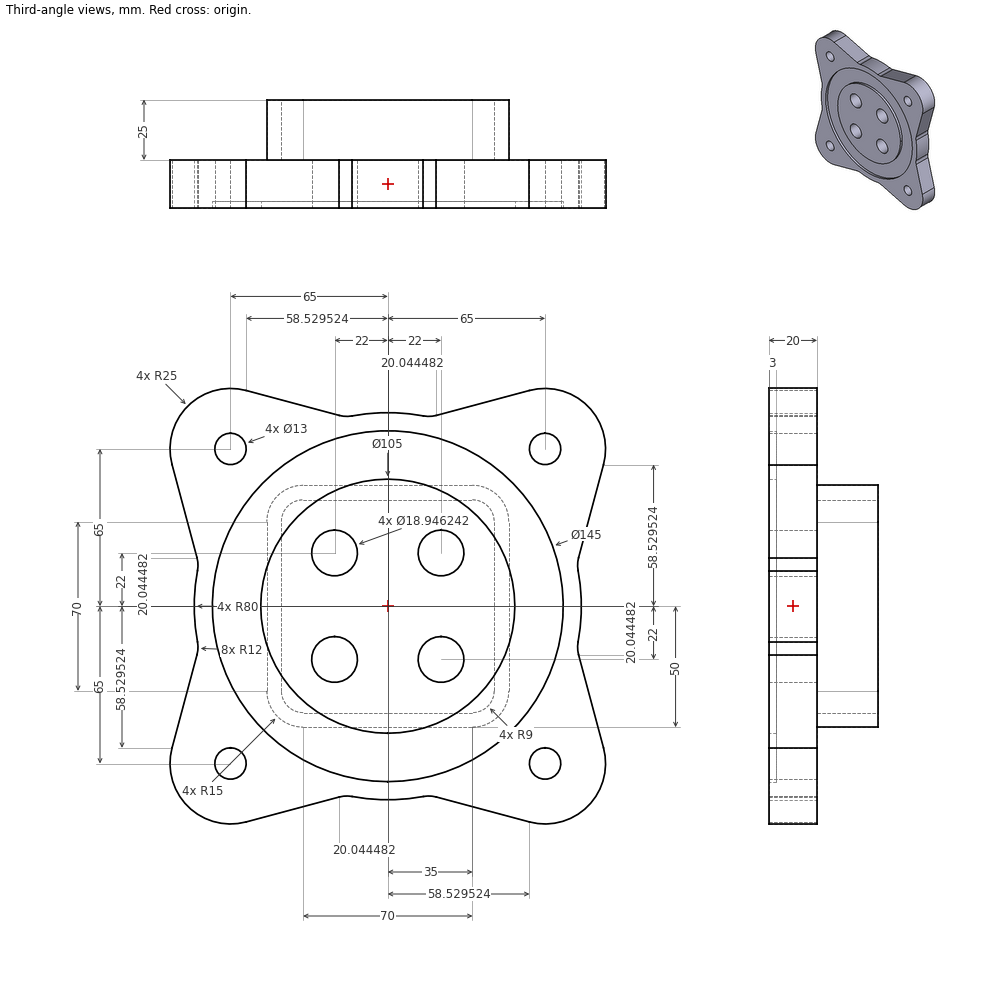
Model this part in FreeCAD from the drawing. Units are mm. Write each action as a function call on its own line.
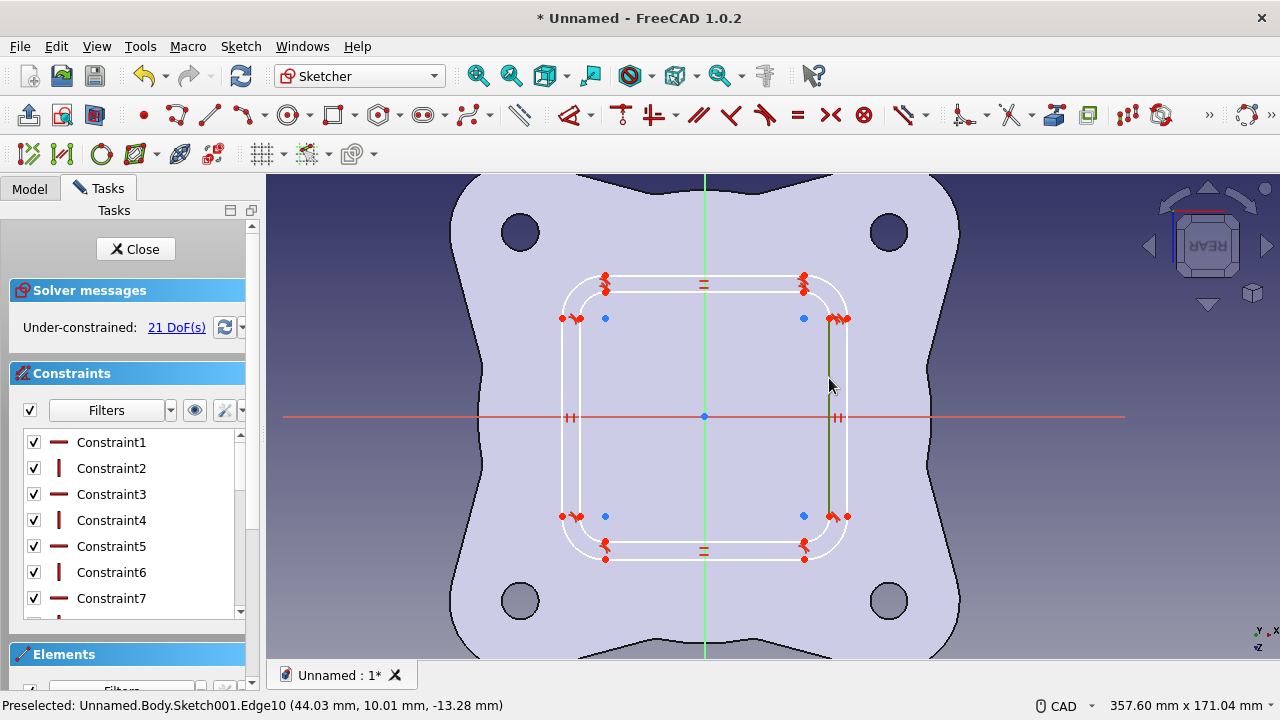
click(816, 539)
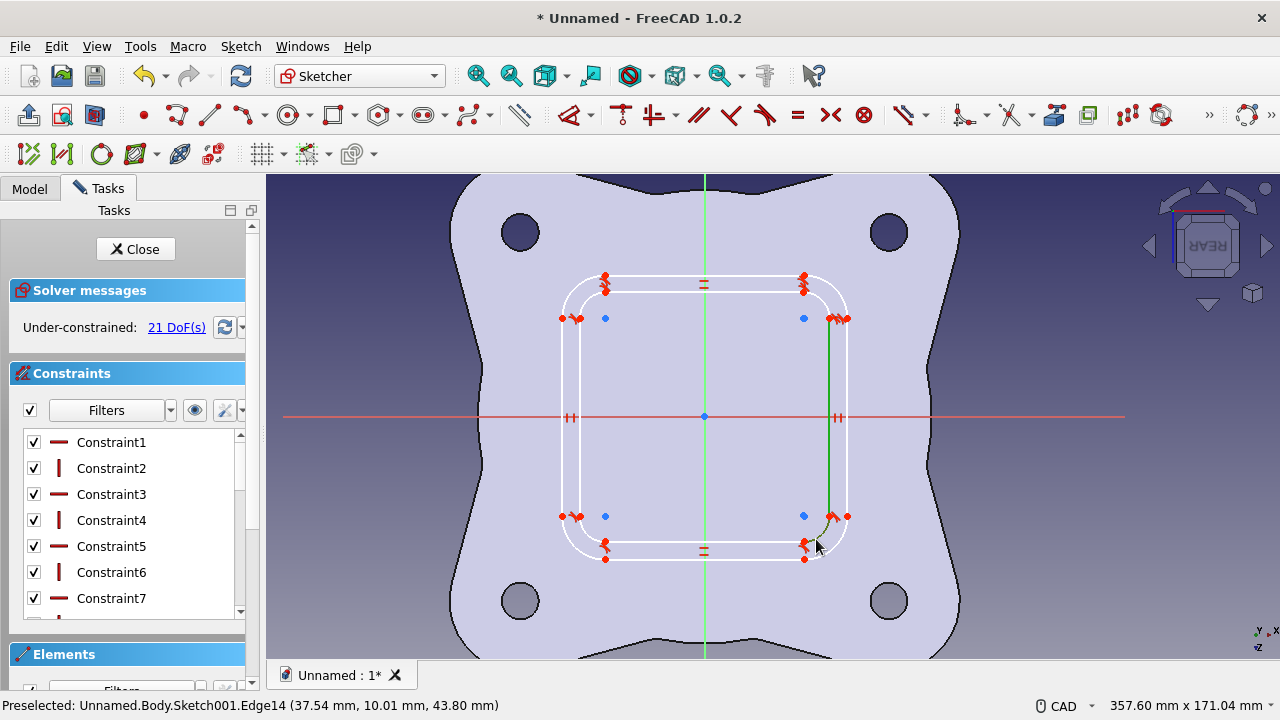
key(t)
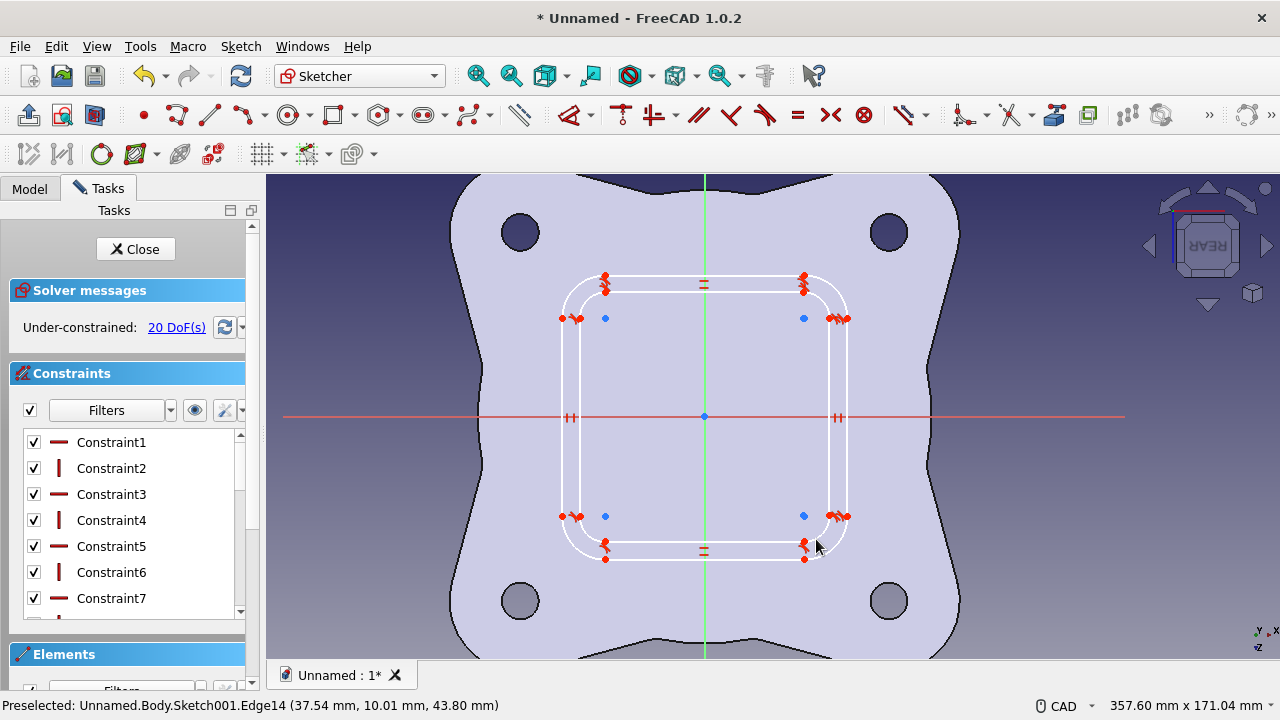
click(744, 542)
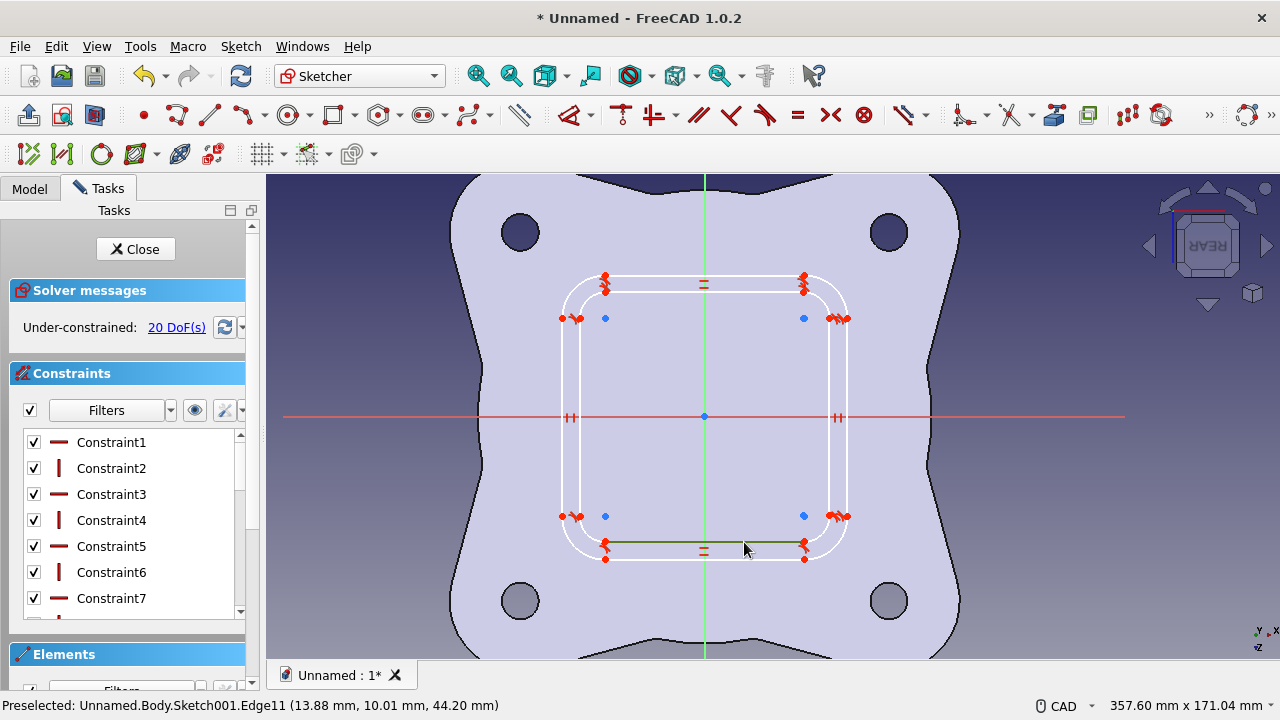
click(816, 539)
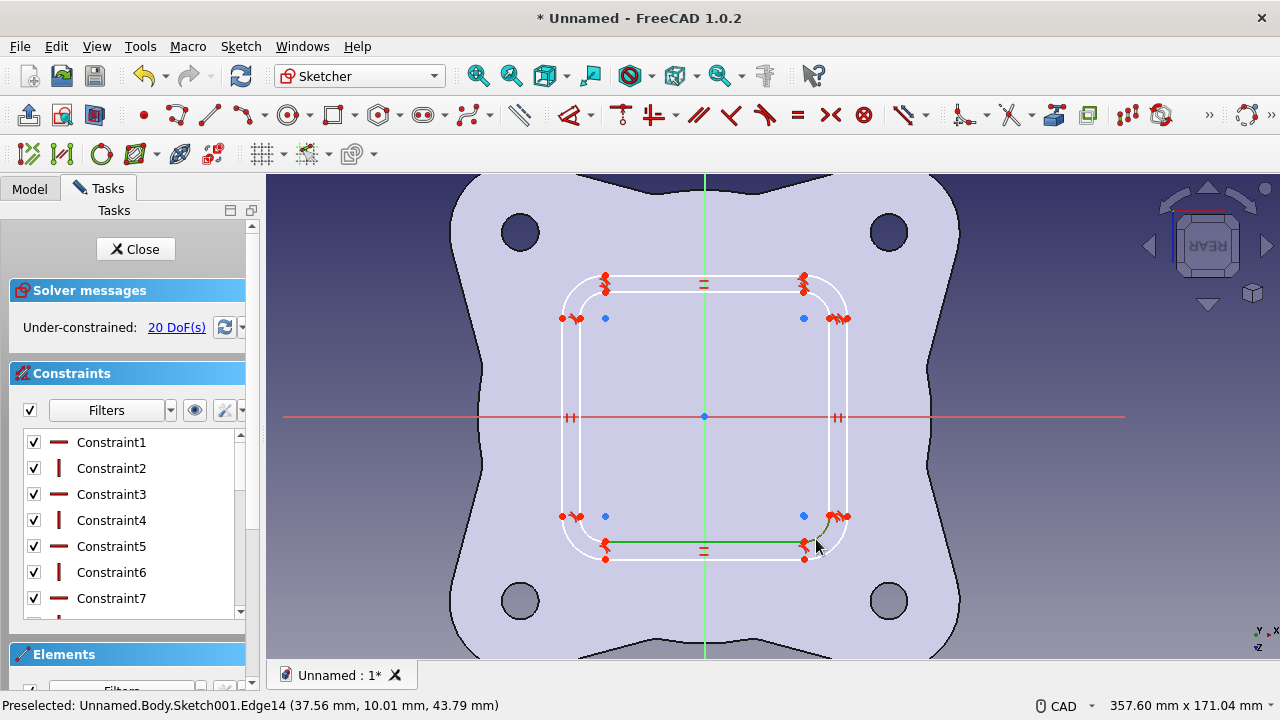
click(765, 116)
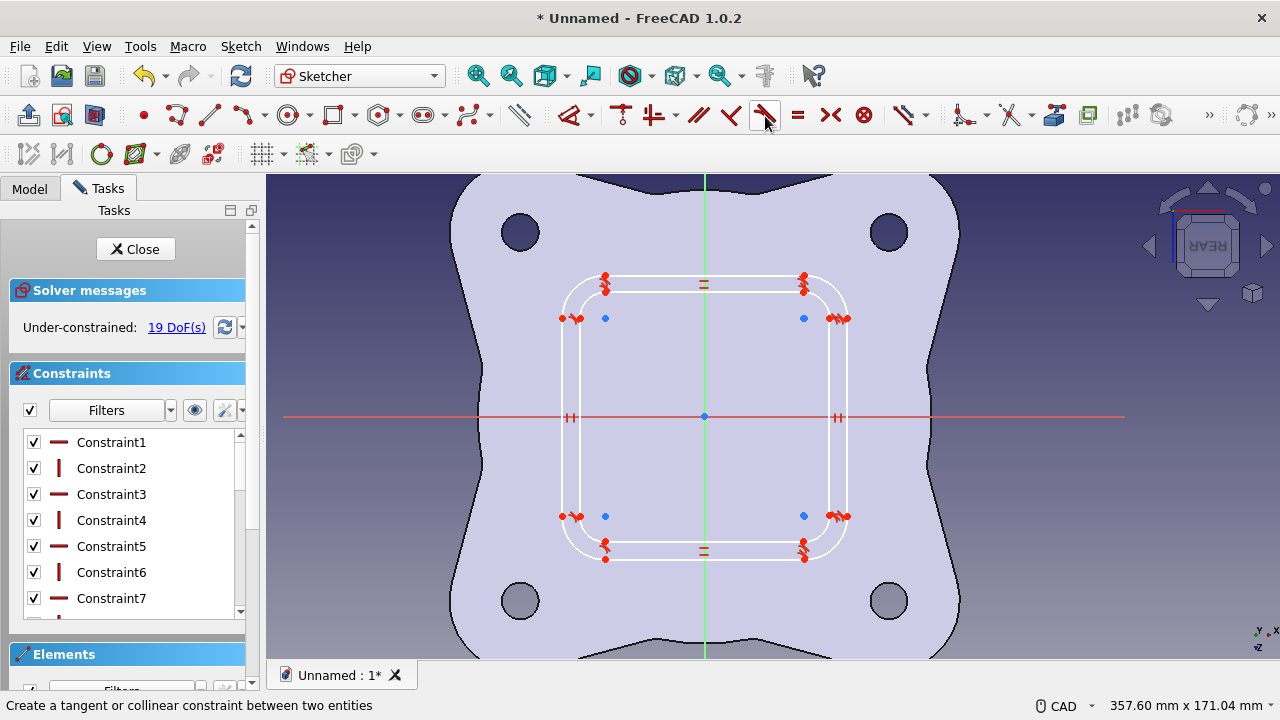
click(744, 542)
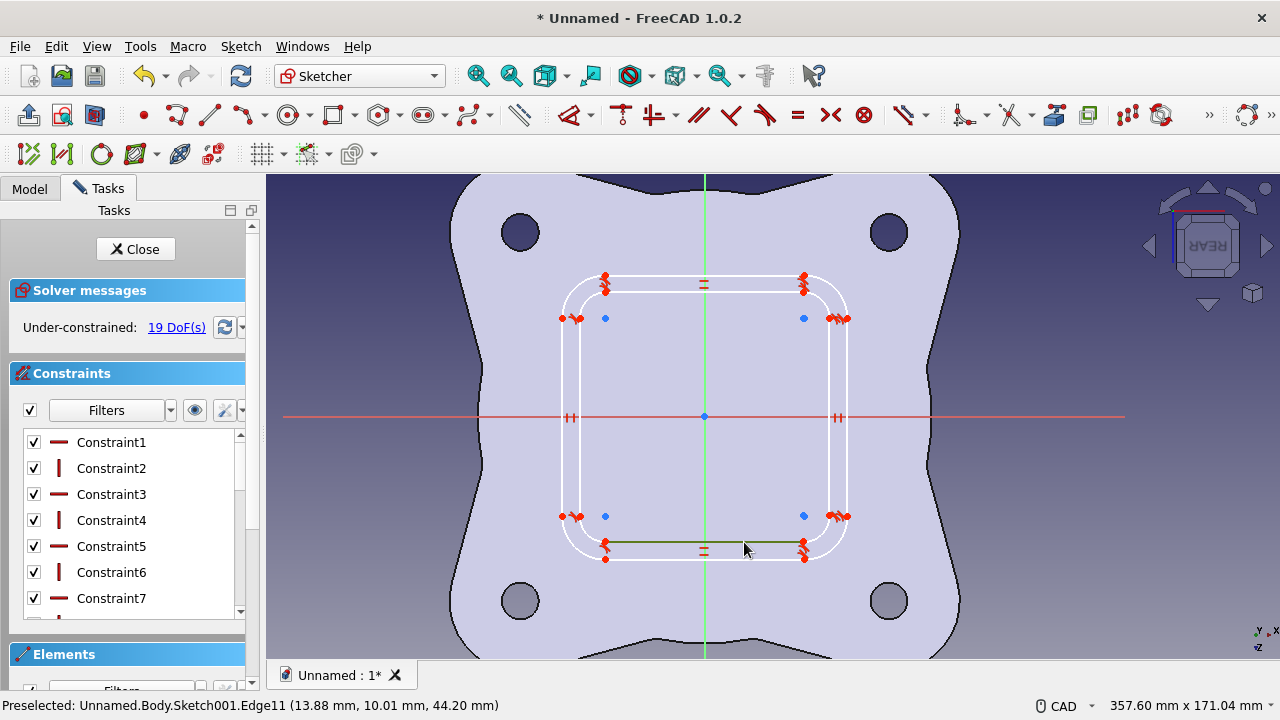
click(583, 528)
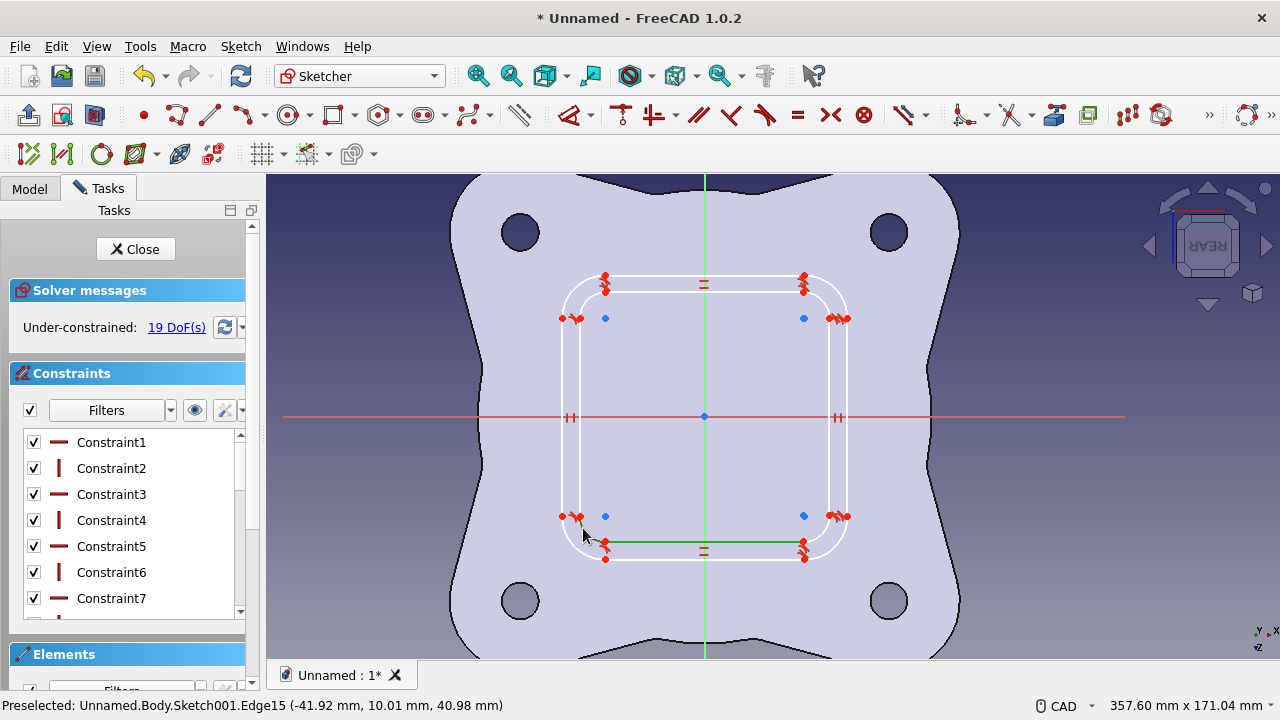
click(765, 116)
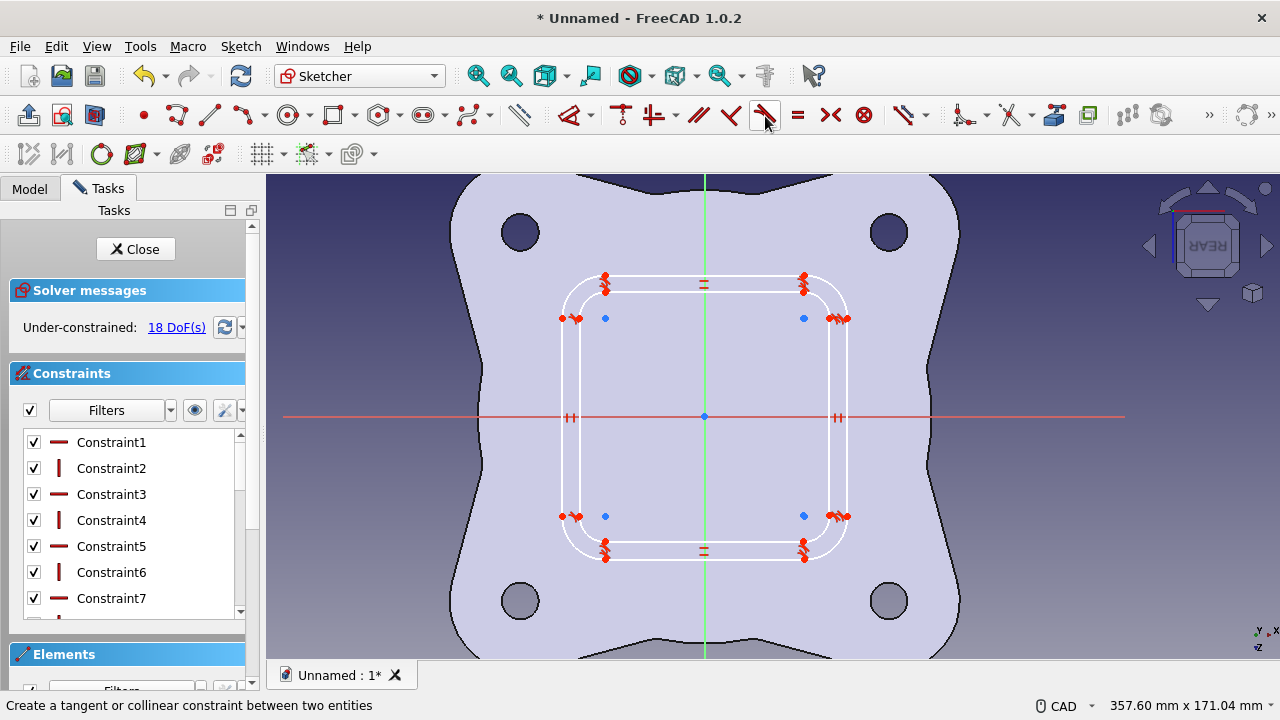
click(580, 457)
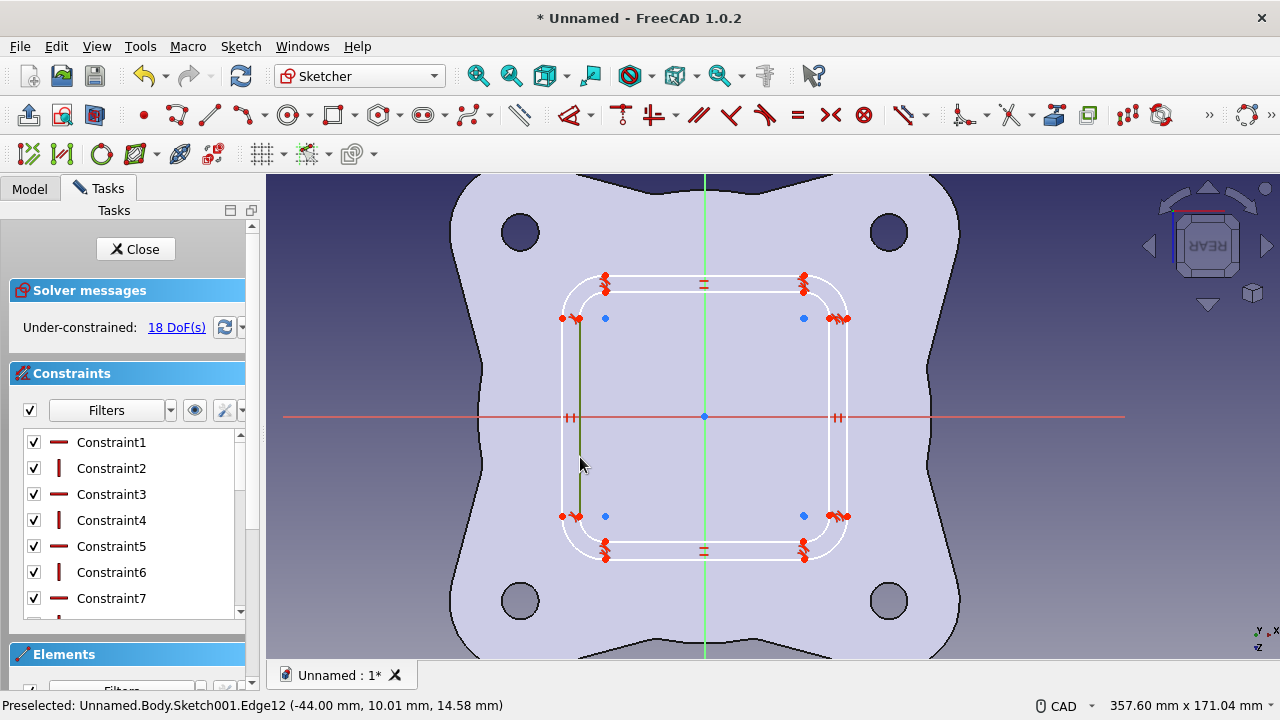
click(583, 528)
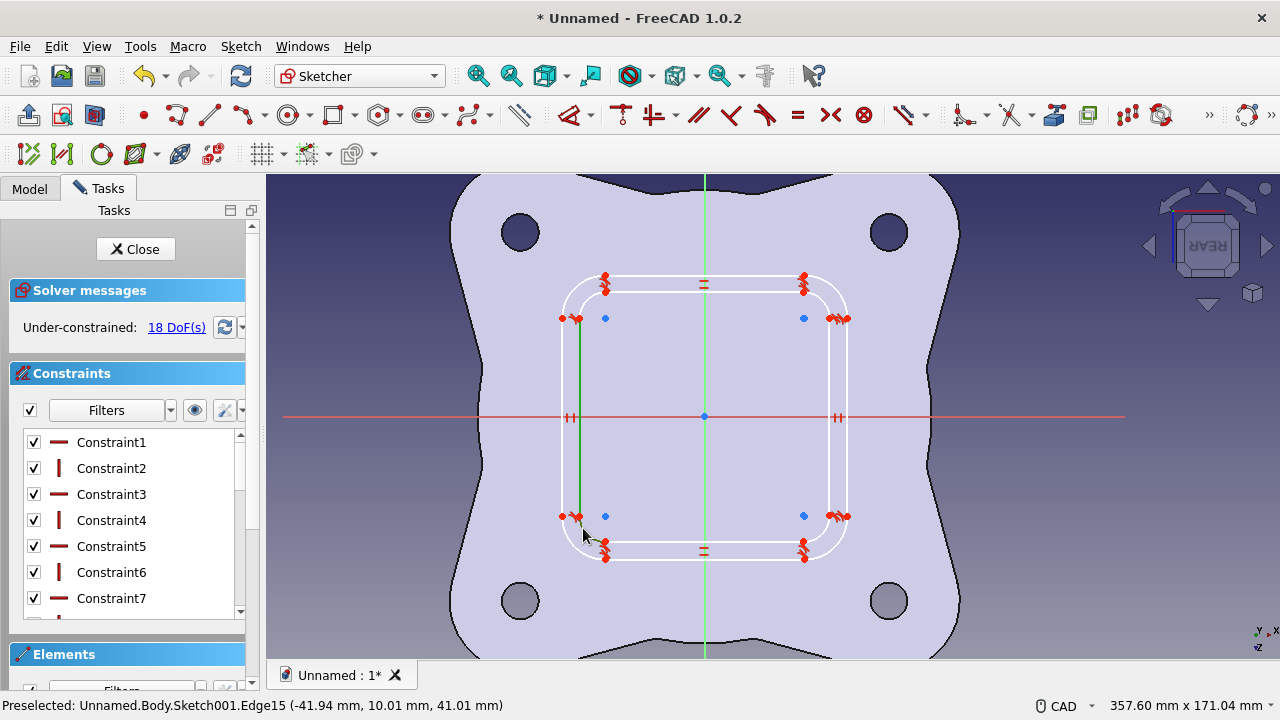
click(765, 116)